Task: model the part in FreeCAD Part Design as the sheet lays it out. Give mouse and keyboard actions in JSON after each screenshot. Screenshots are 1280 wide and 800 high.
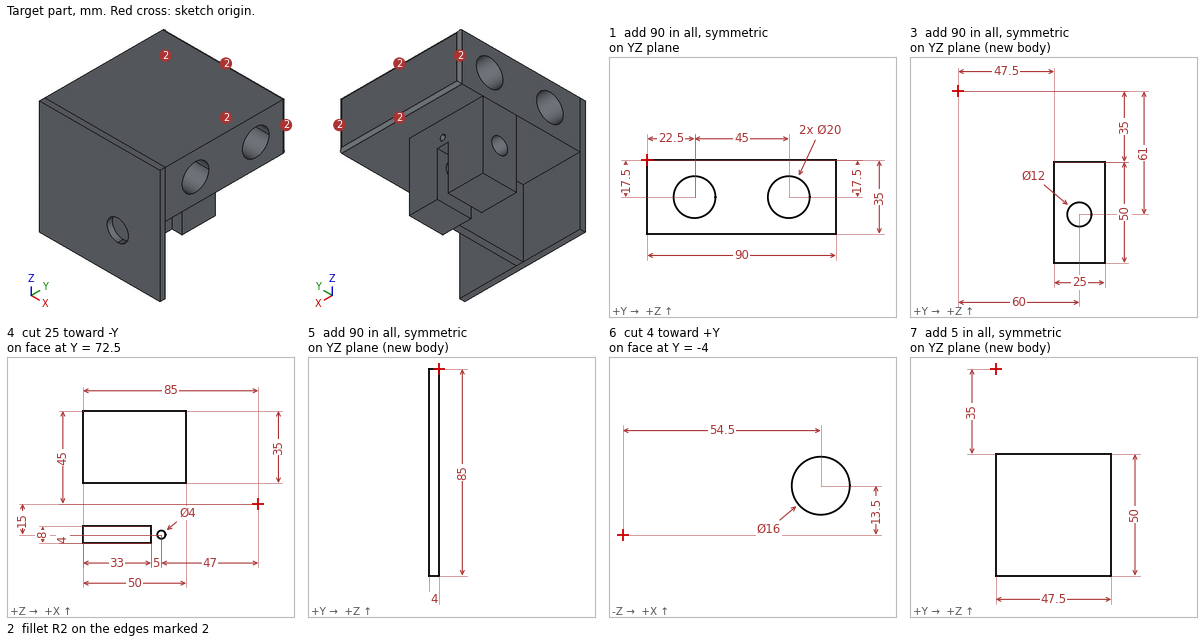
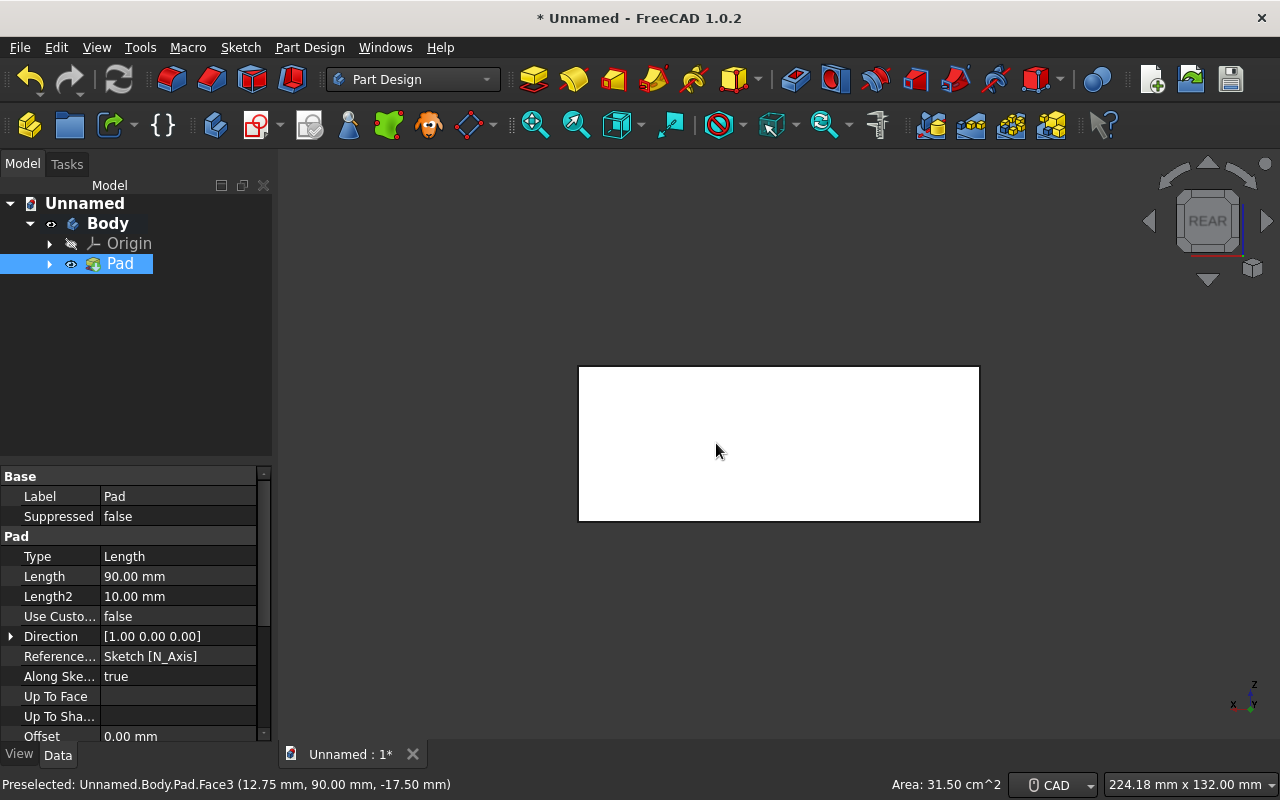
{"action": "left_click", "coordinate": [172, 80]}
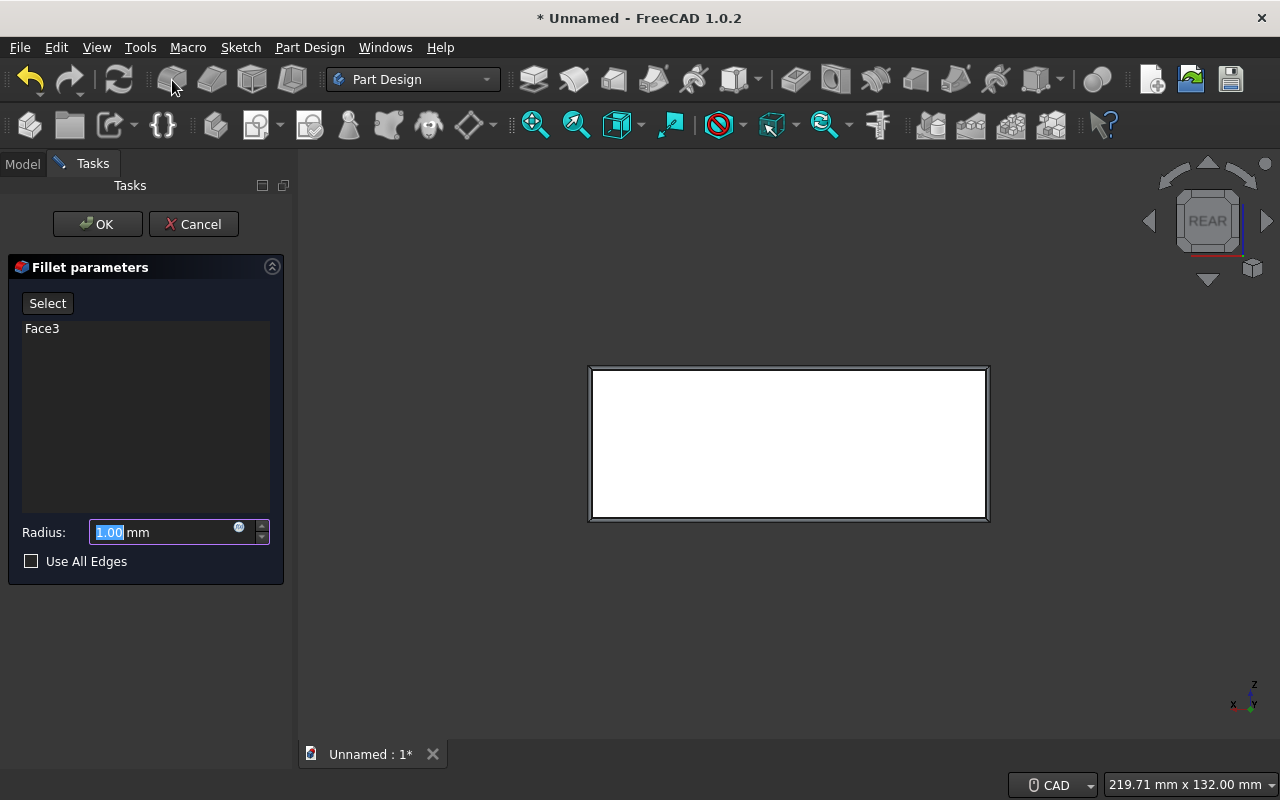
{"action": "type", "text": "2"}
{"action": "key", "text": "Tab"}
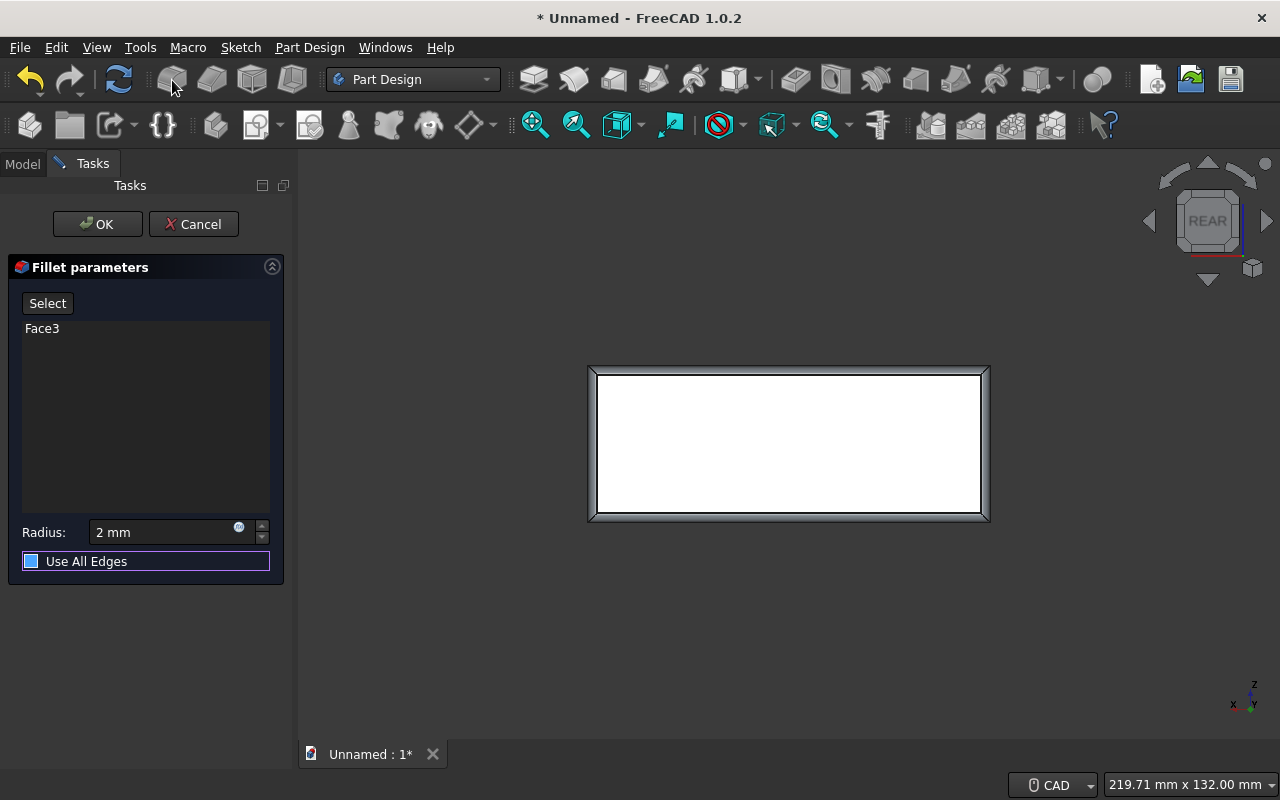
{"action": "left_click", "coordinate": [98, 224]}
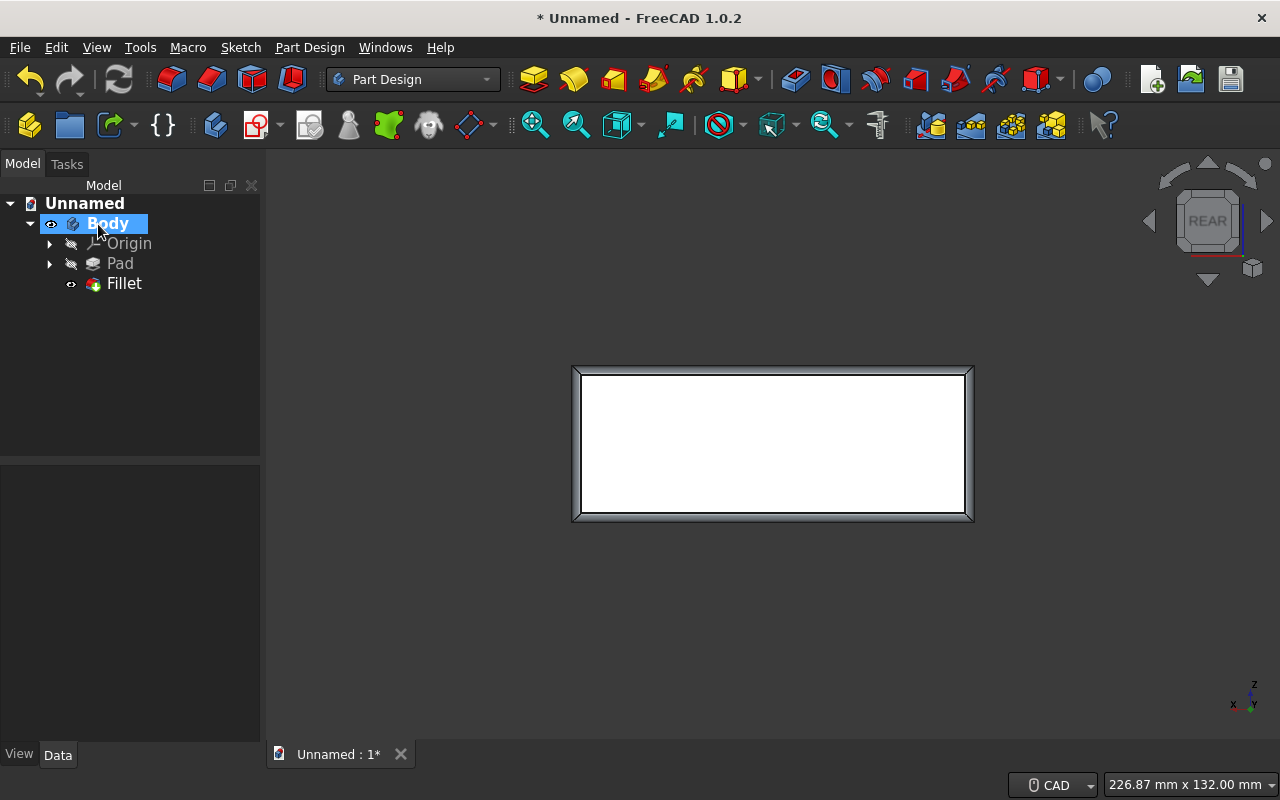
{"action": "left_click", "coordinate": [536, 126]}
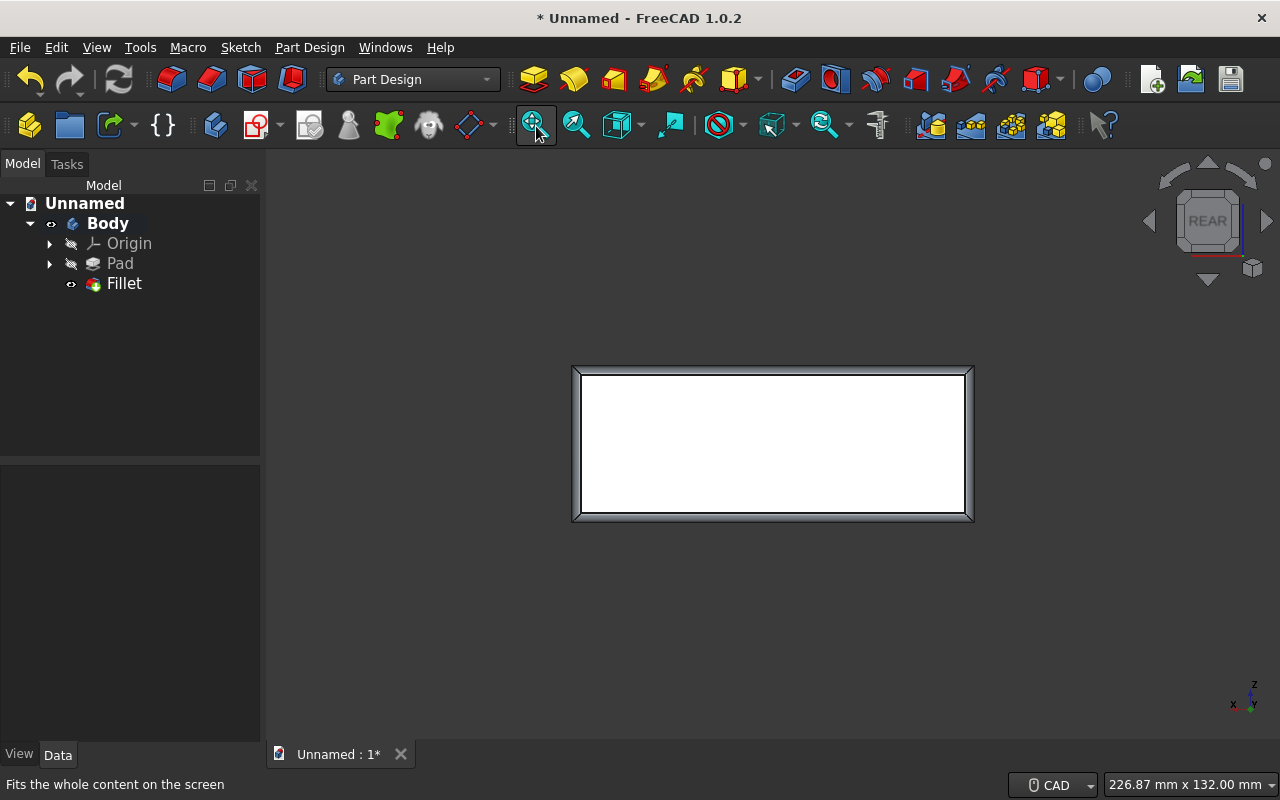
{"action": "left_click", "coordinate": [216, 126]}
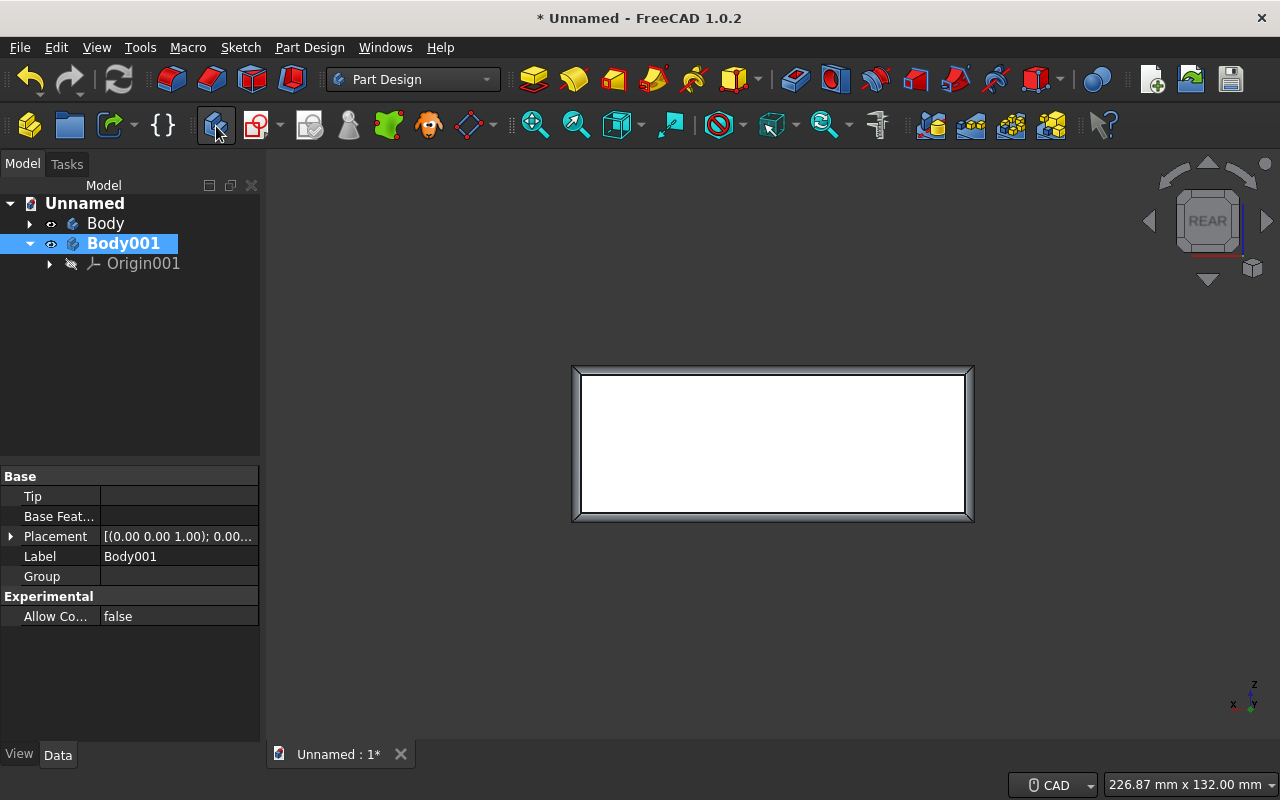
{"action": "left_click", "coordinate": [306, 699]}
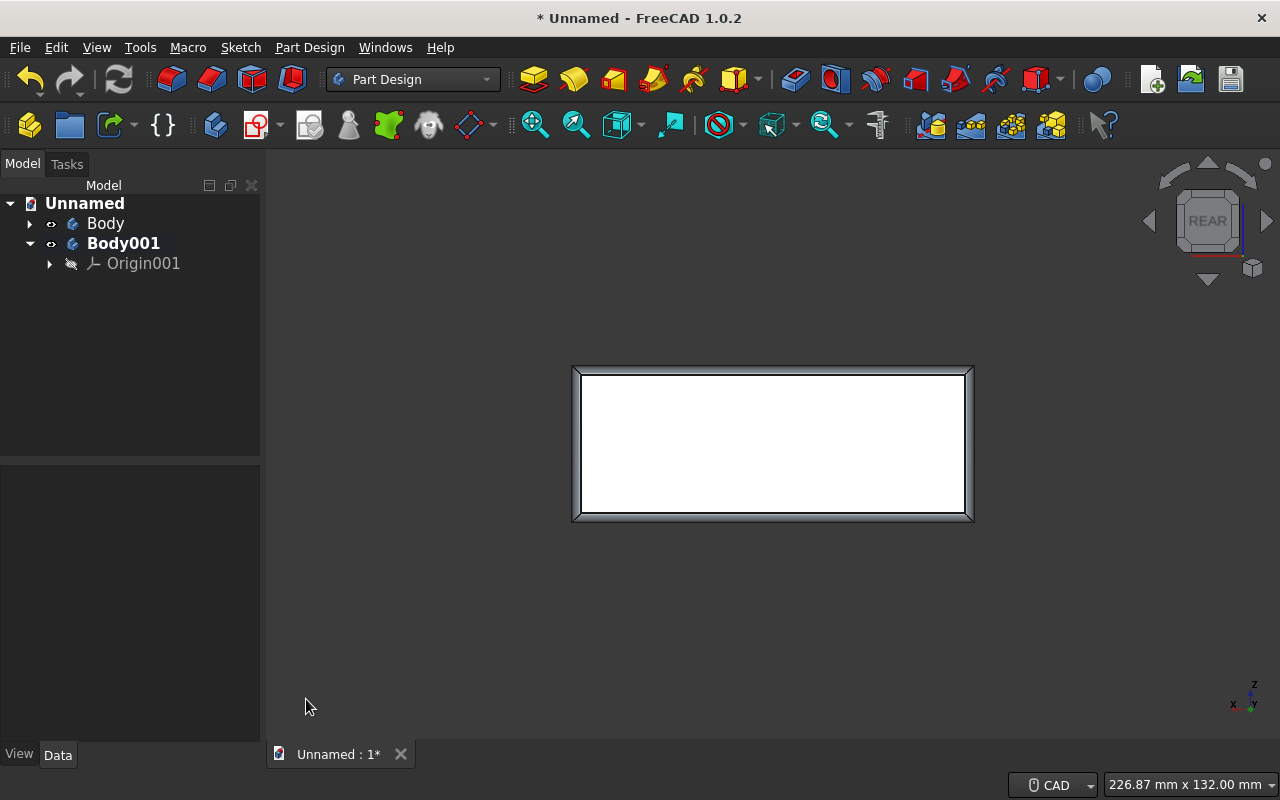
{"action": "left_click", "coordinate": [256, 126]}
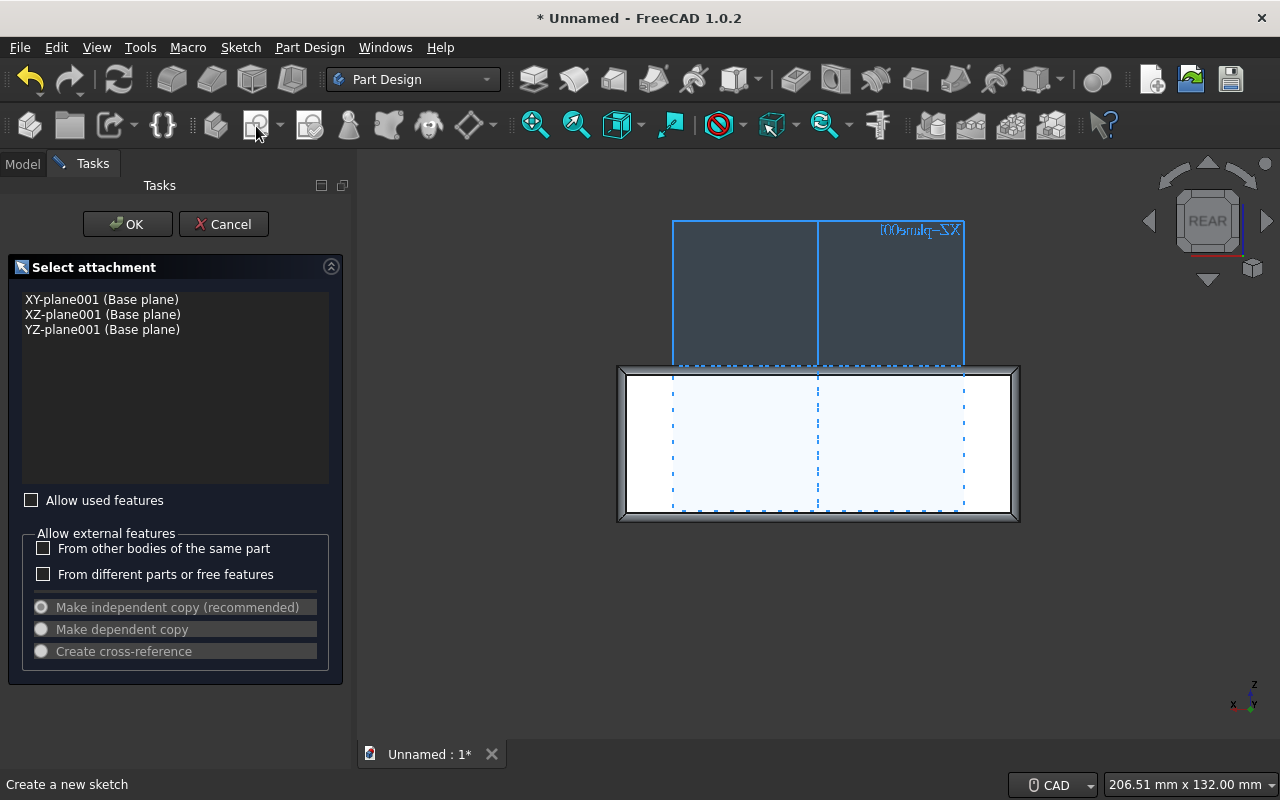
{"action": "left_click", "coordinate": [82, 330]}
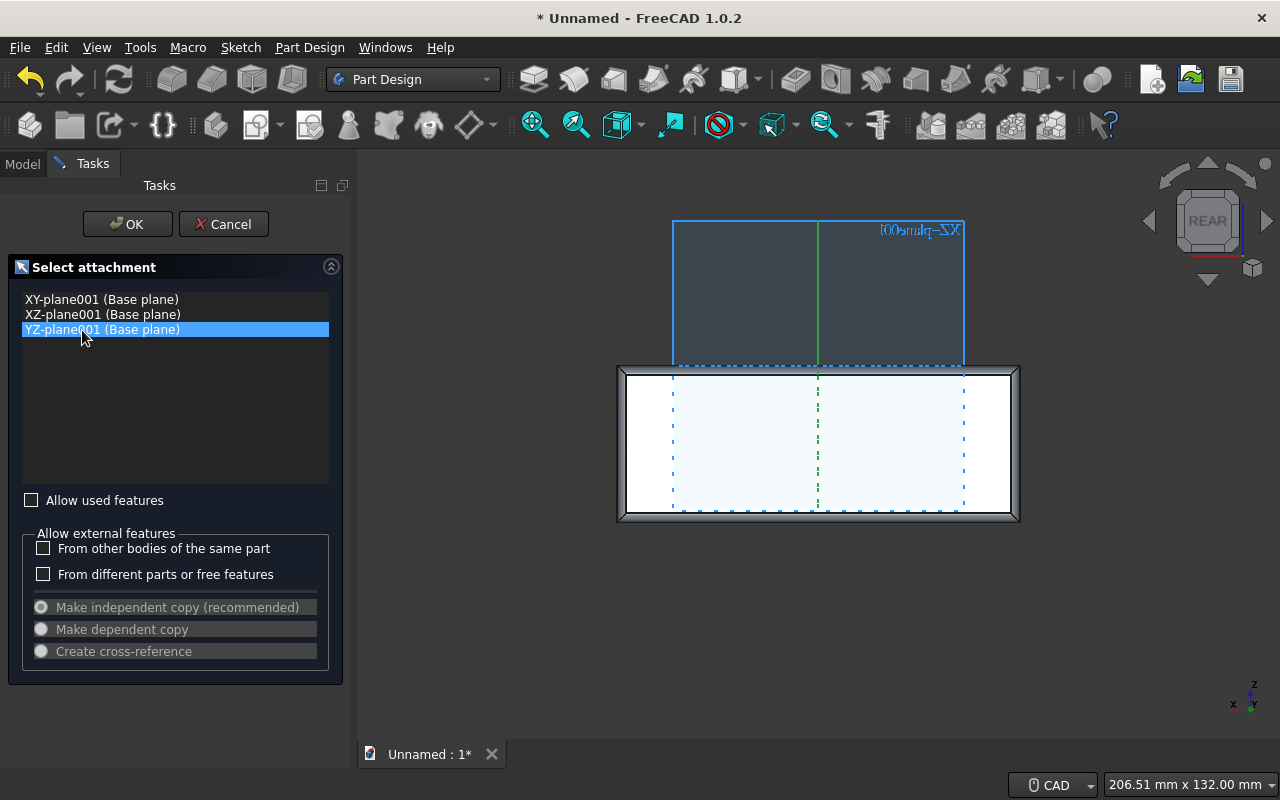
{"action": "left_click", "coordinate": [128, 224]}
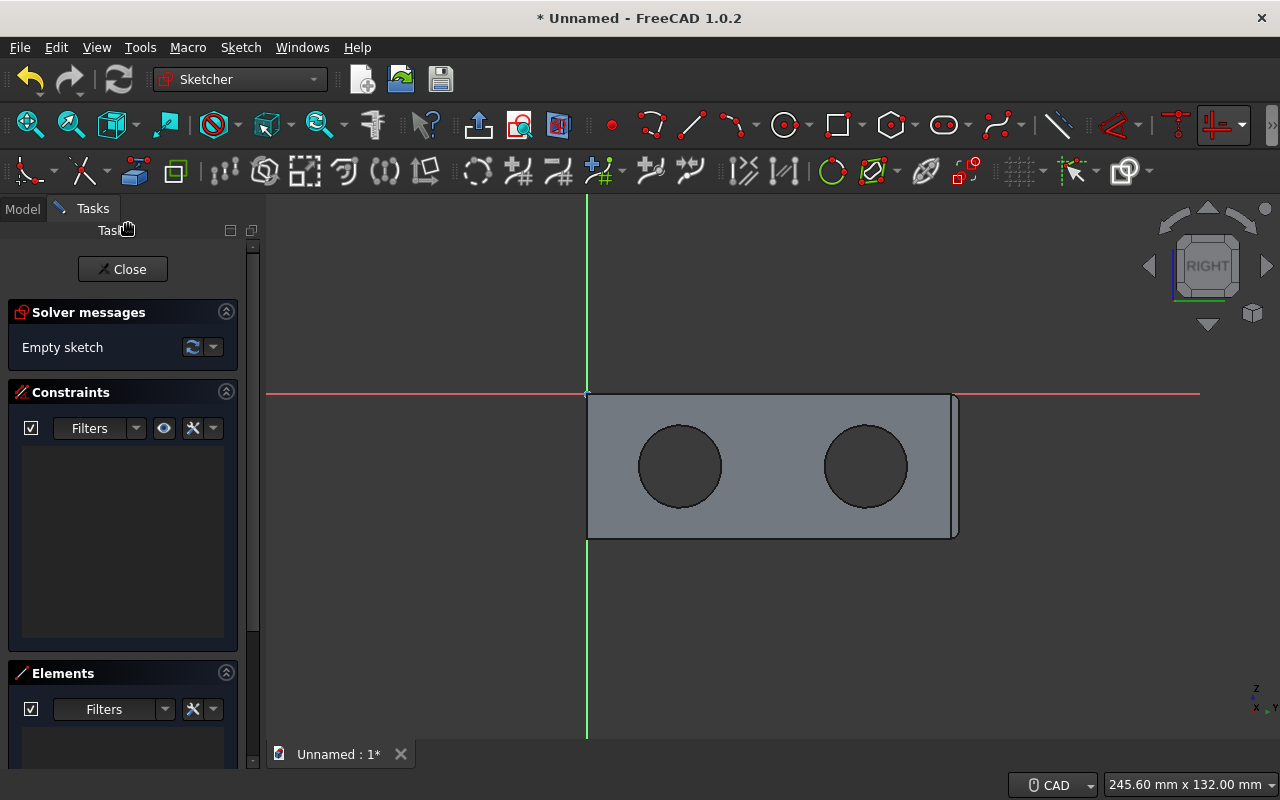
{"action": "scroll", "coordinate": [558, 222], "scroll_direction": "down", "scroll_amount": 1}